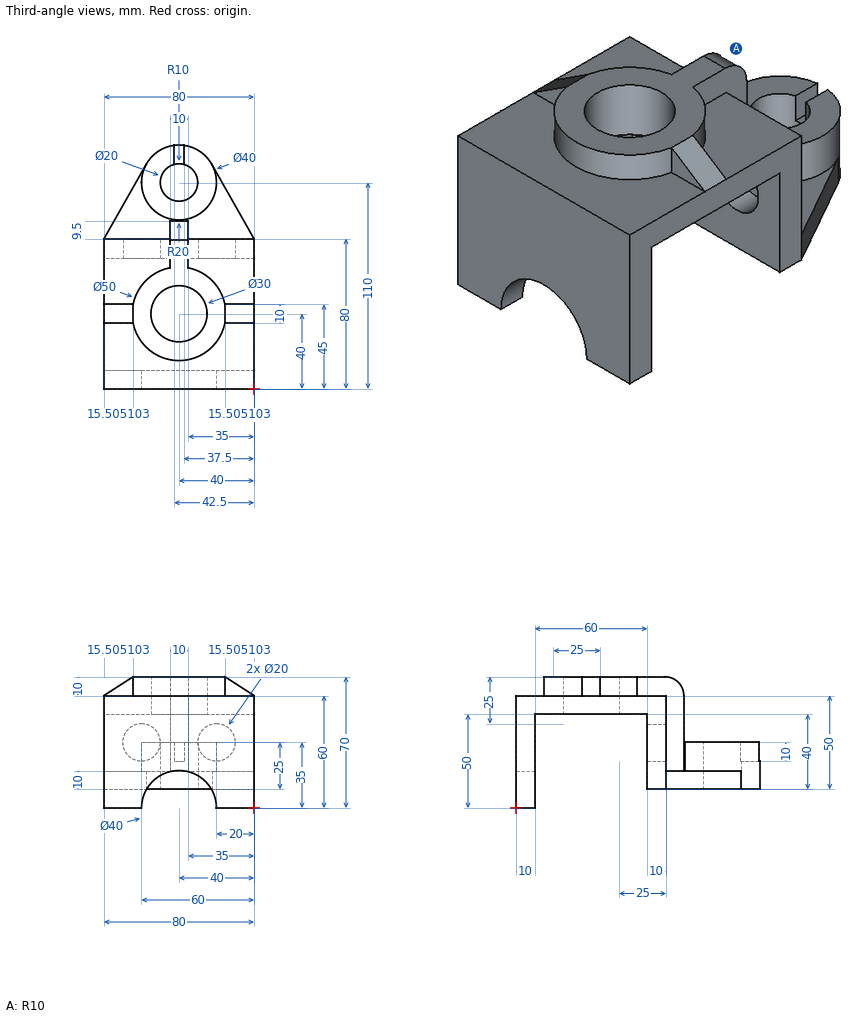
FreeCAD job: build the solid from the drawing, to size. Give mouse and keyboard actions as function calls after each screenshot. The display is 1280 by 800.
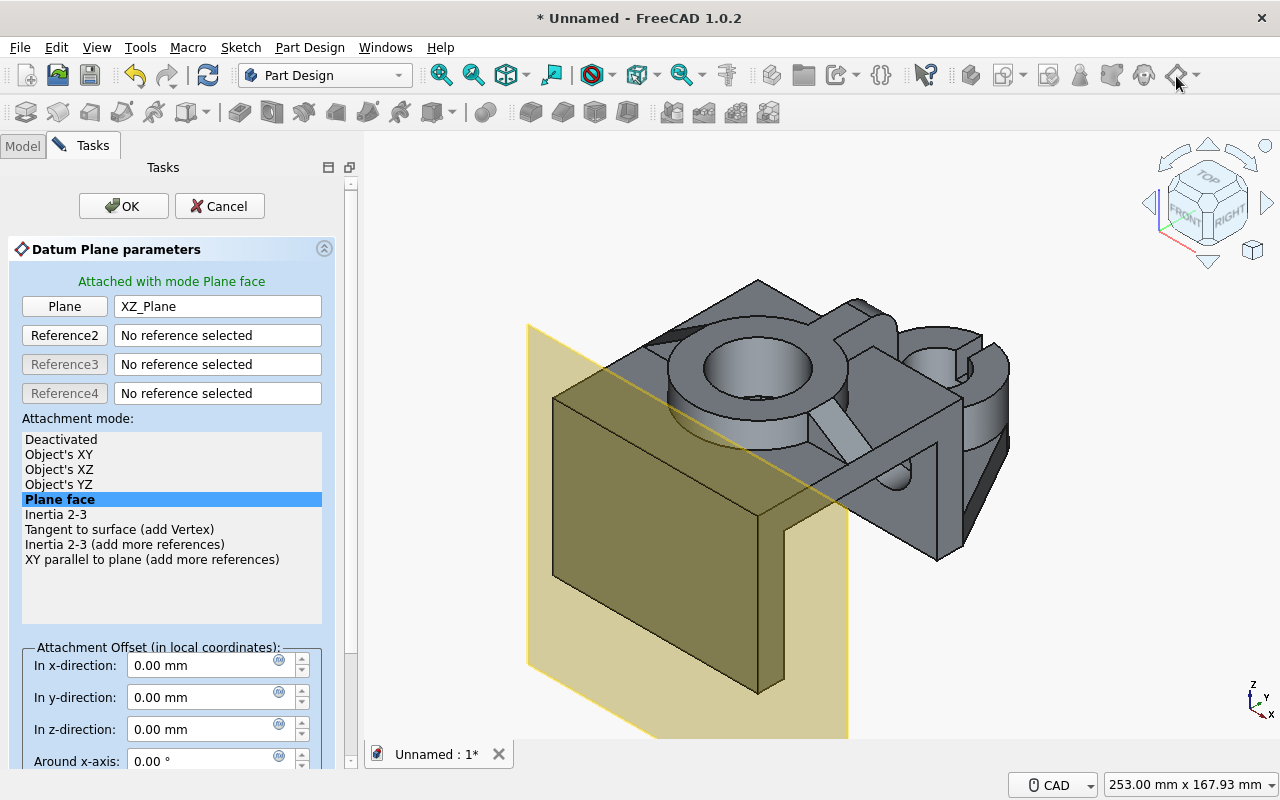
triple_click(210, 729)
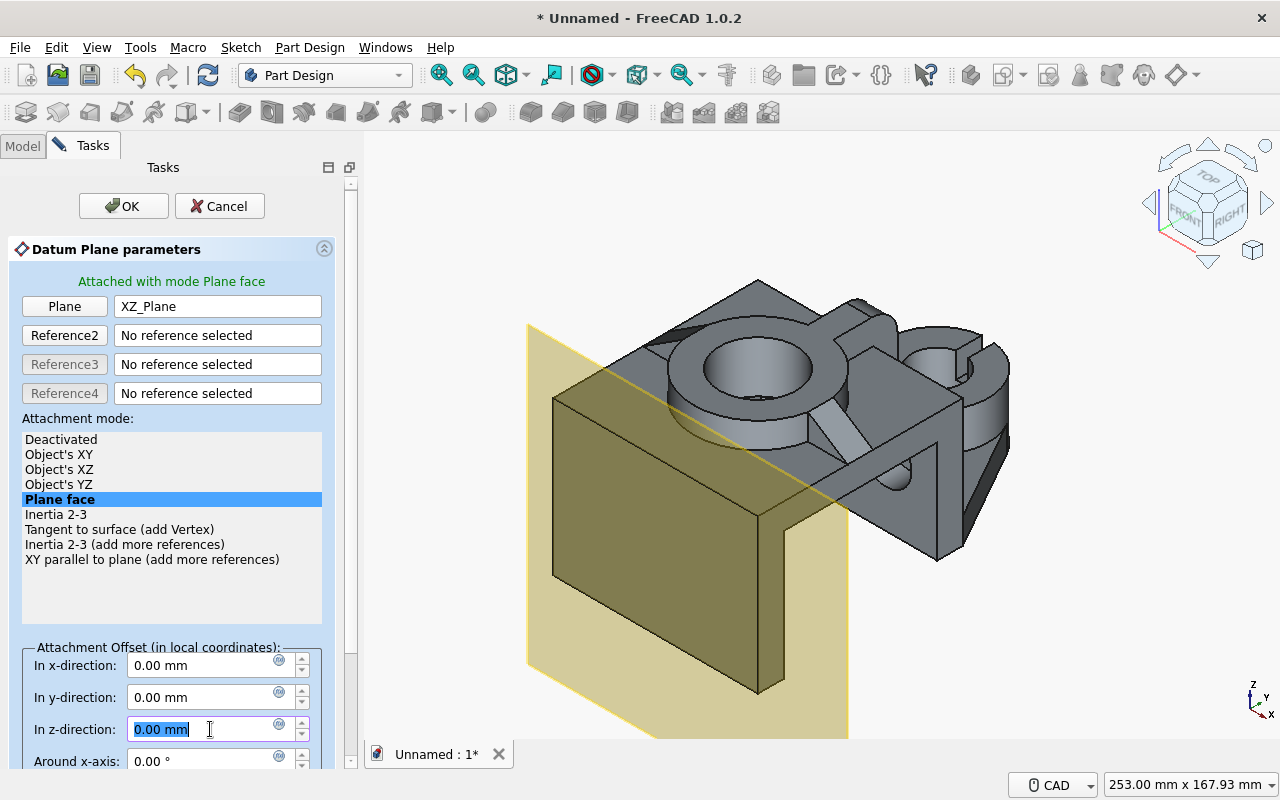
text(-10)
key(Tab)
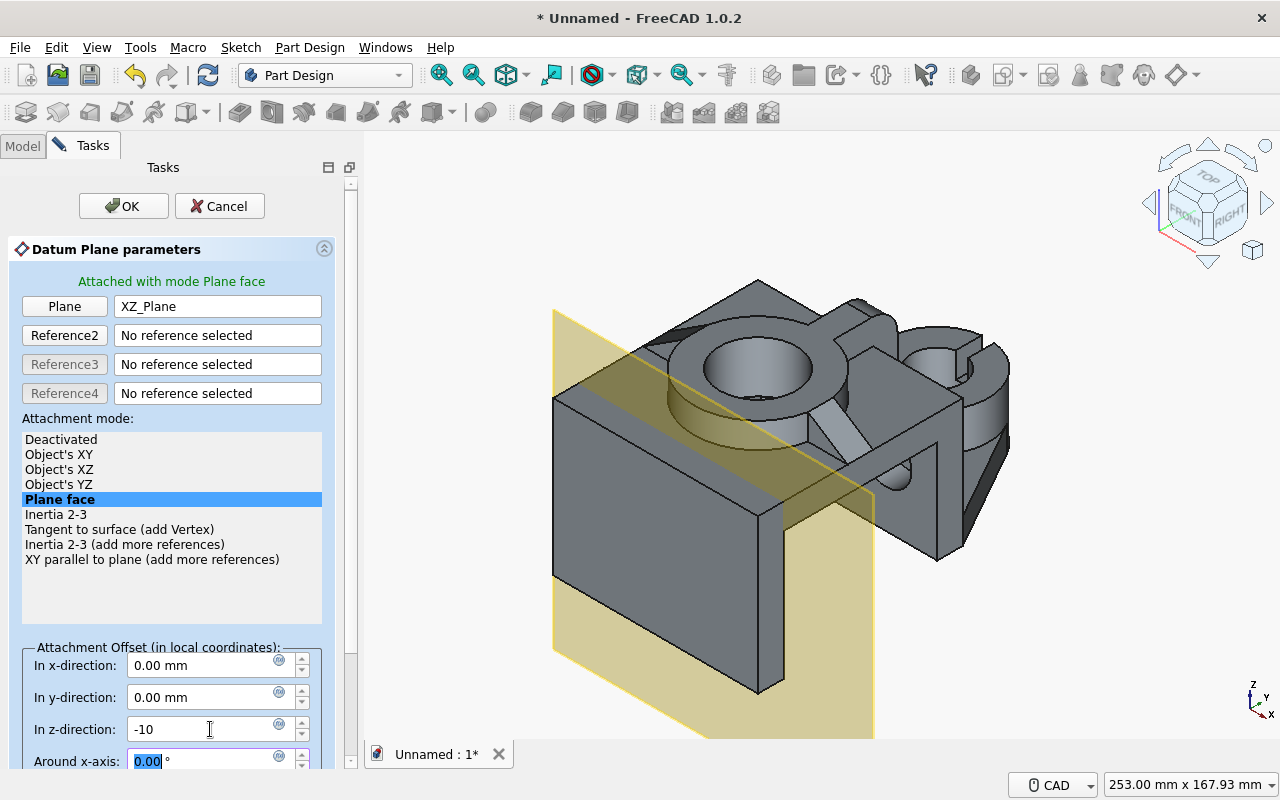
click(124, 206)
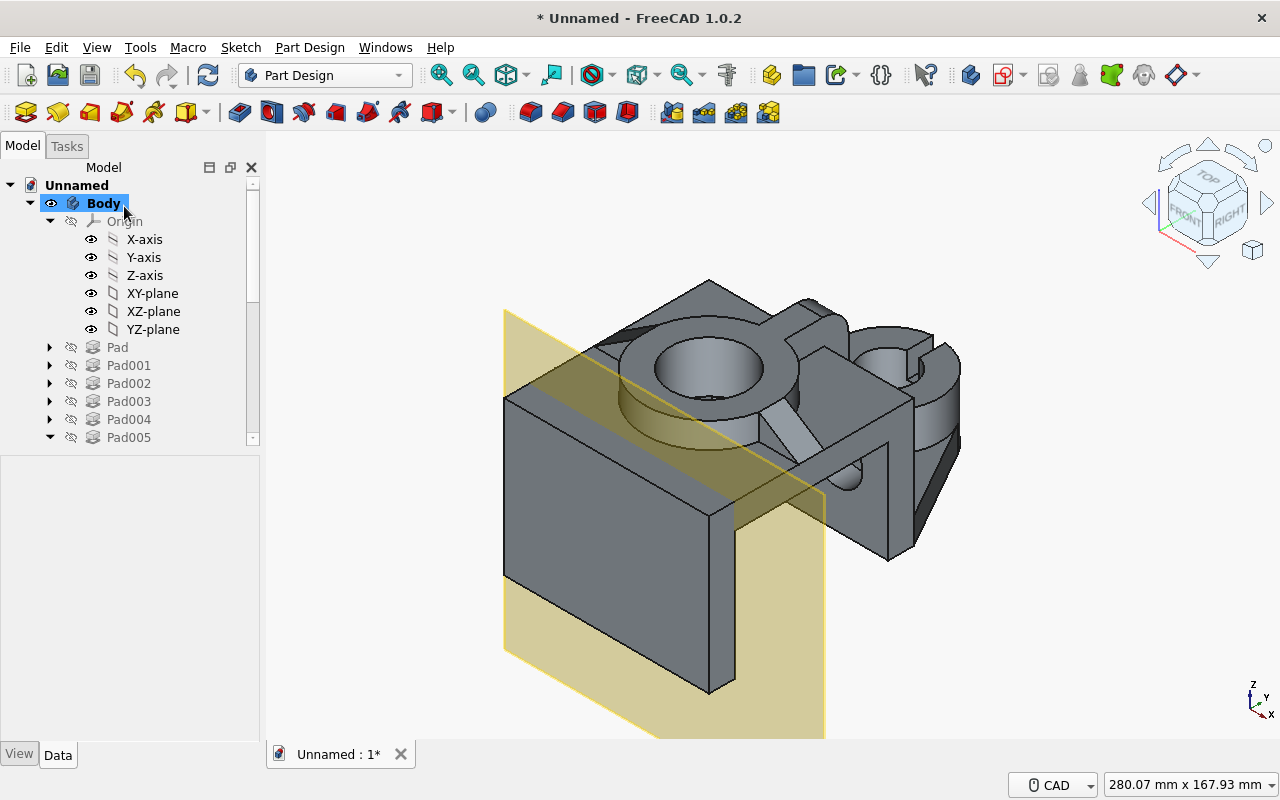
scroll(100, 307, down, 3)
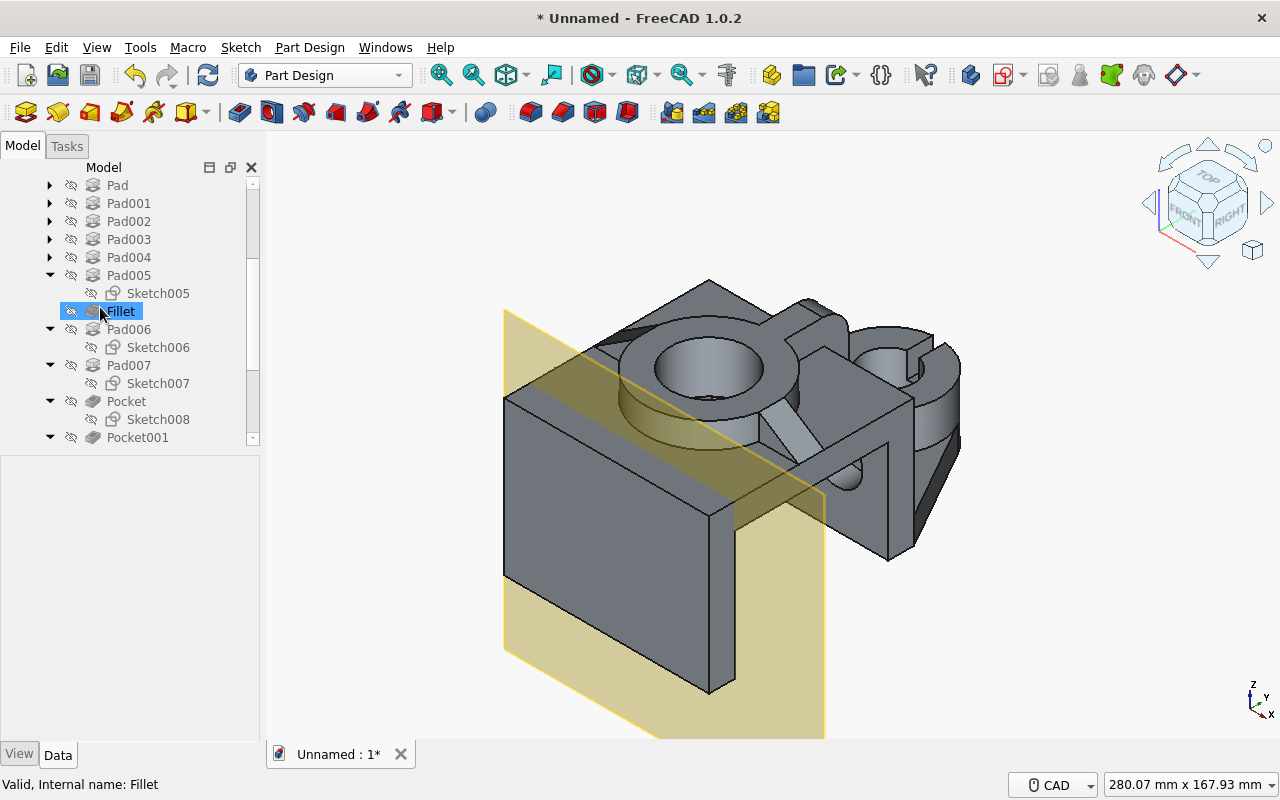
scroll(140, 307, up, 15)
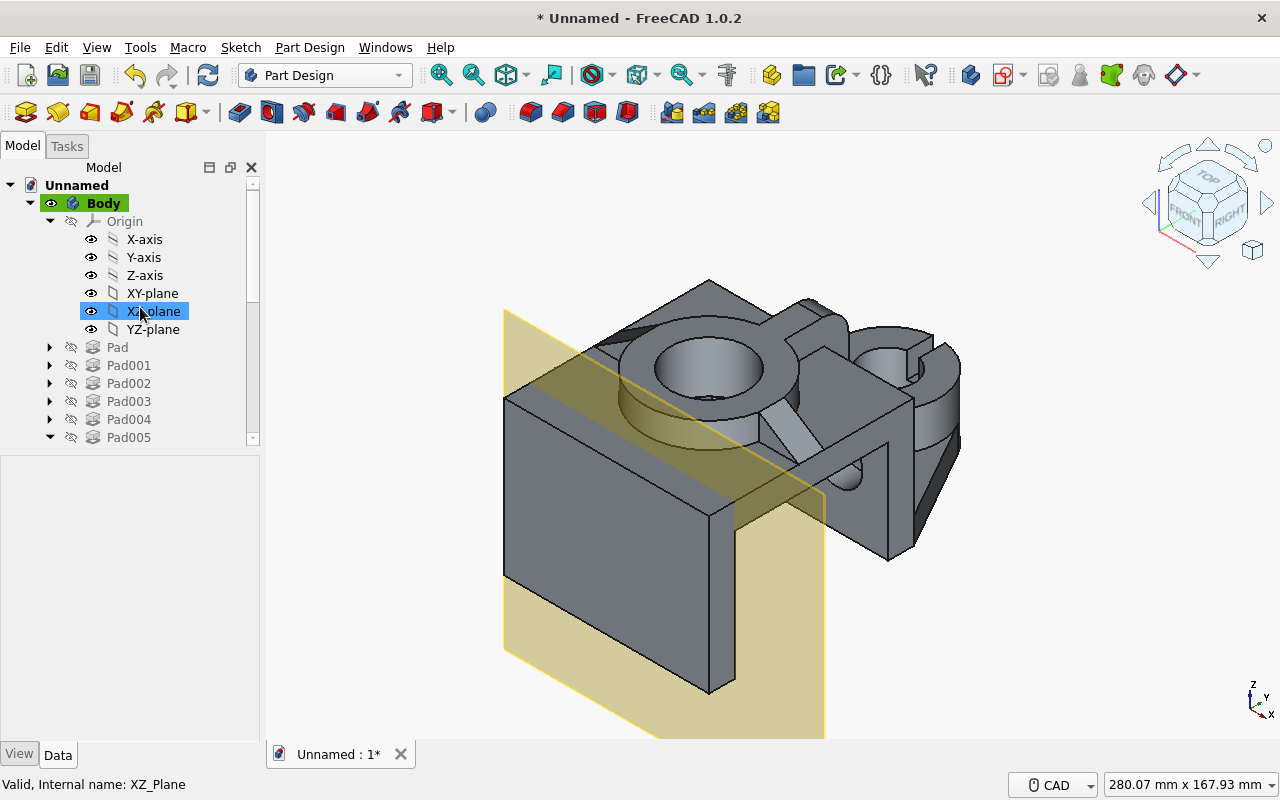
scroll(100, 307, down, 6)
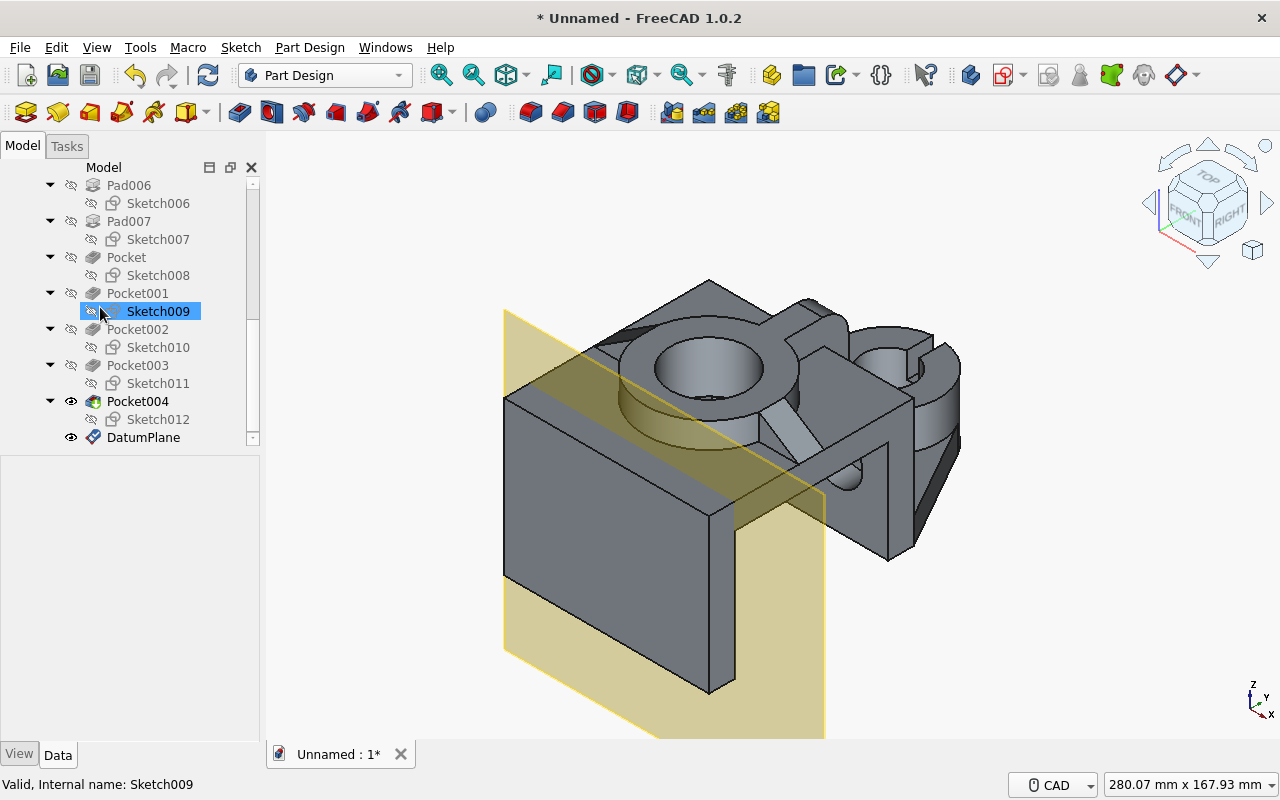
click(116, 437)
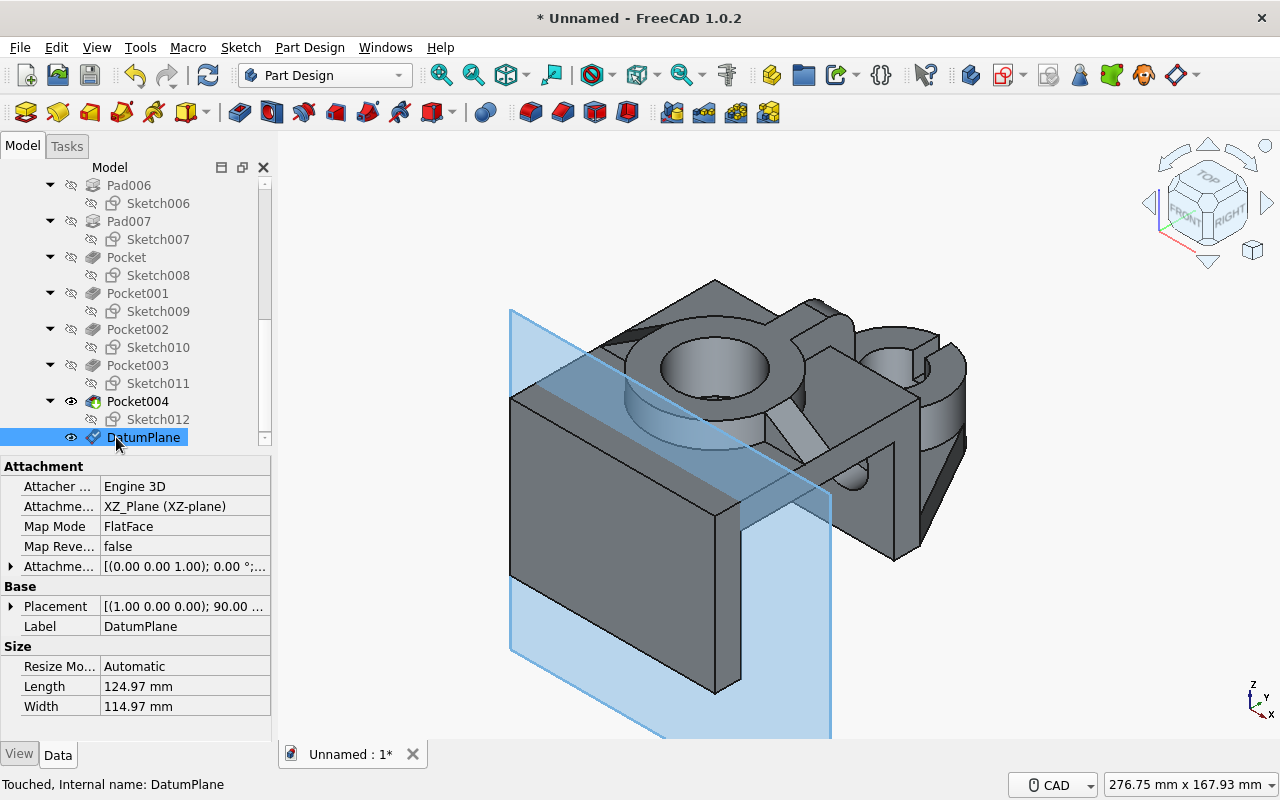
click(1004, 76)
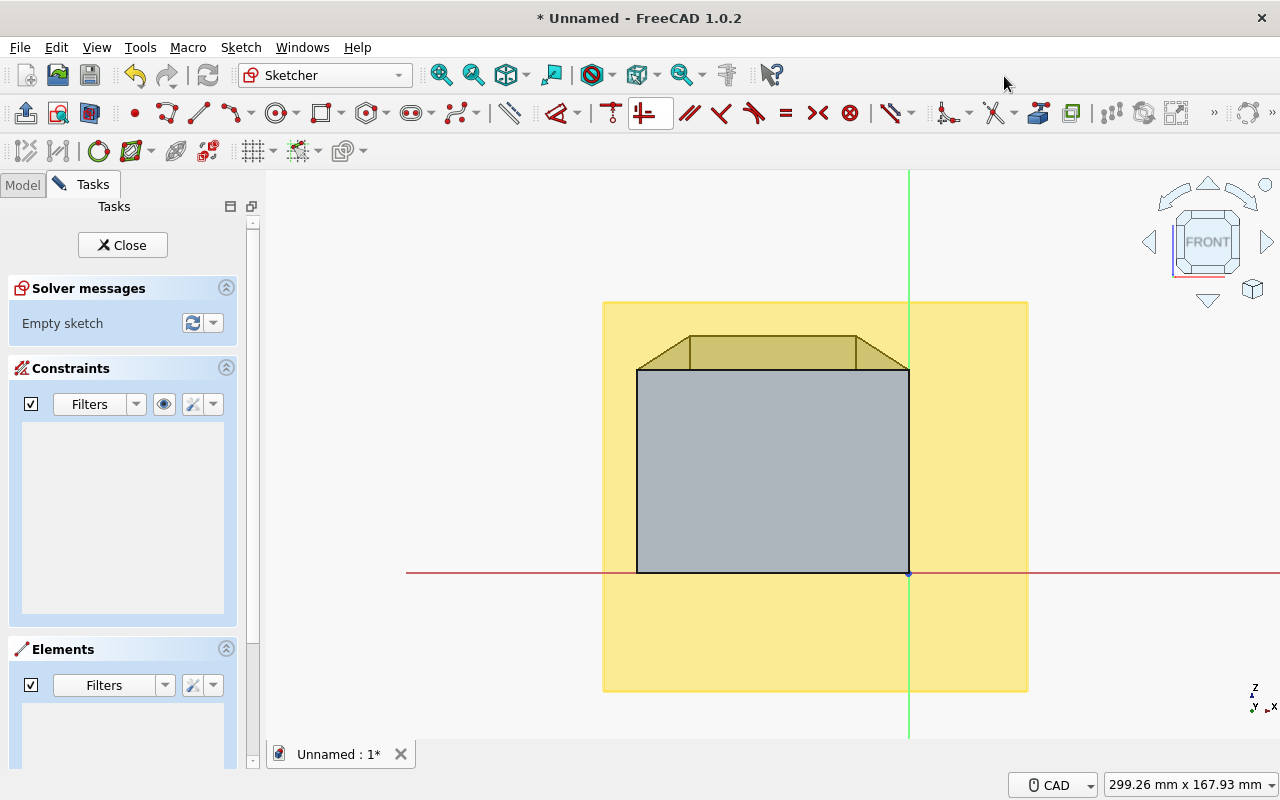
click(90, 114)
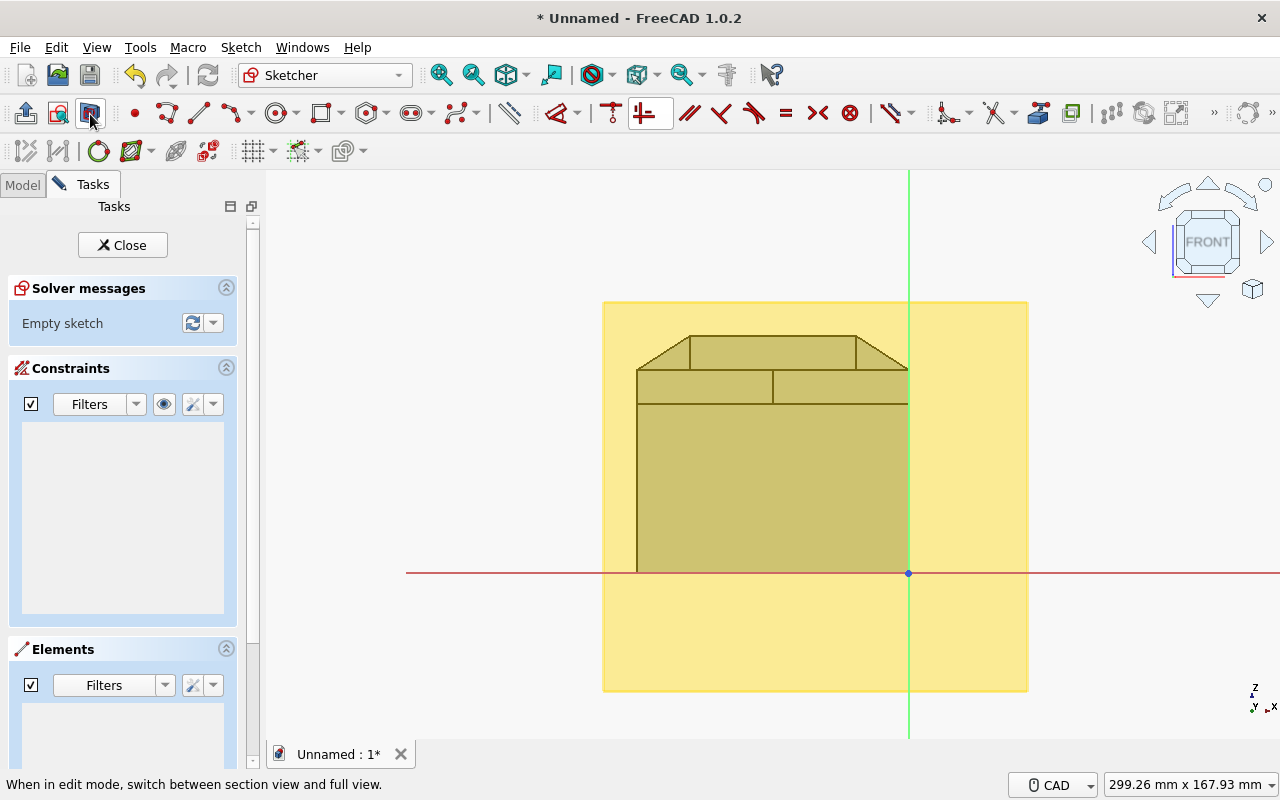
scroll(866, 642, up, 5)